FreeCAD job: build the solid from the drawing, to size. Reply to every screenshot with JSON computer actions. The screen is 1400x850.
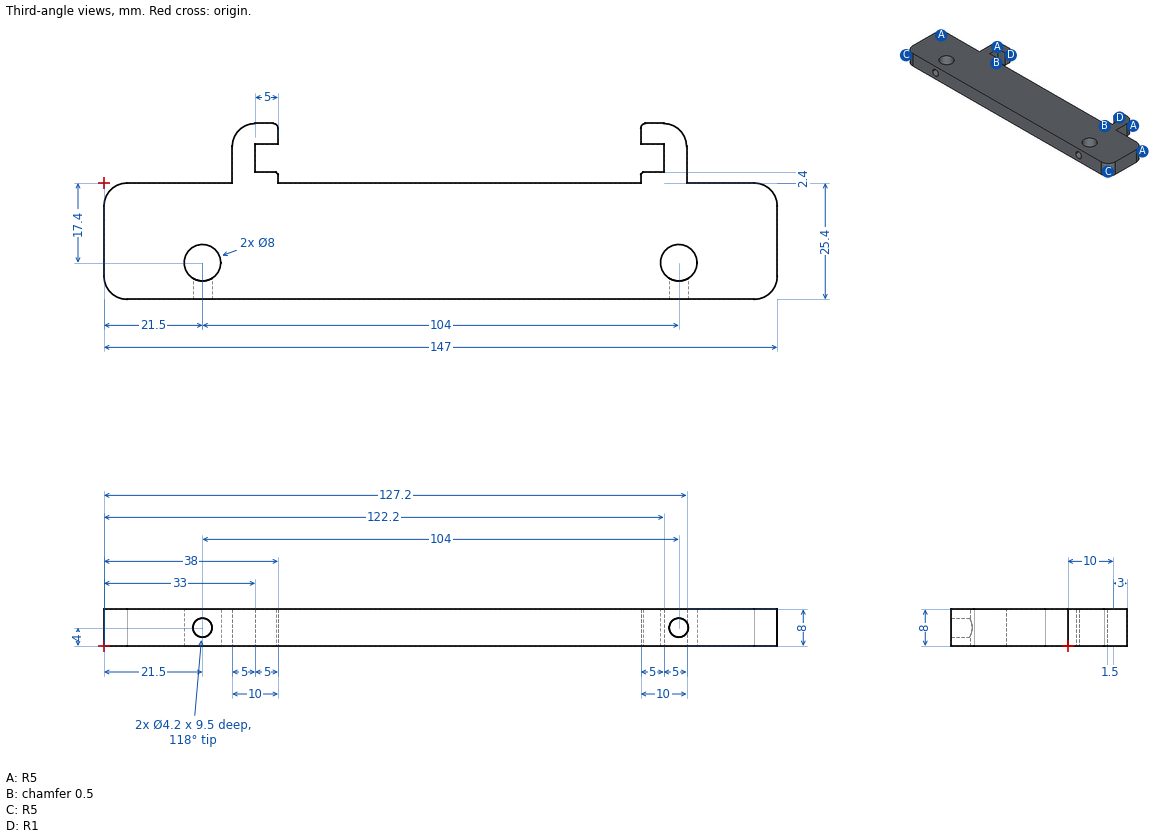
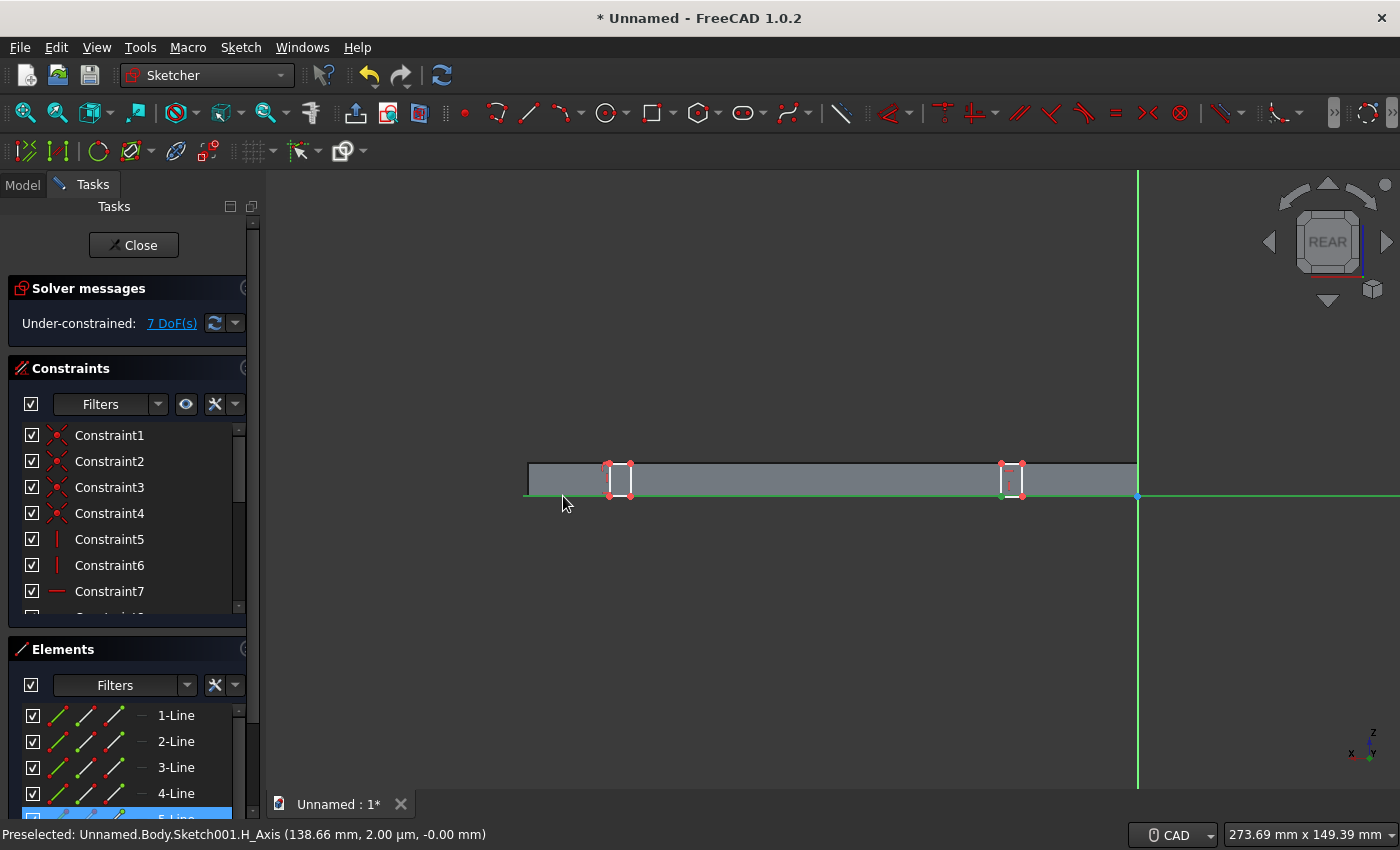
{"action": "left_click", "coordinate": [944, 114]}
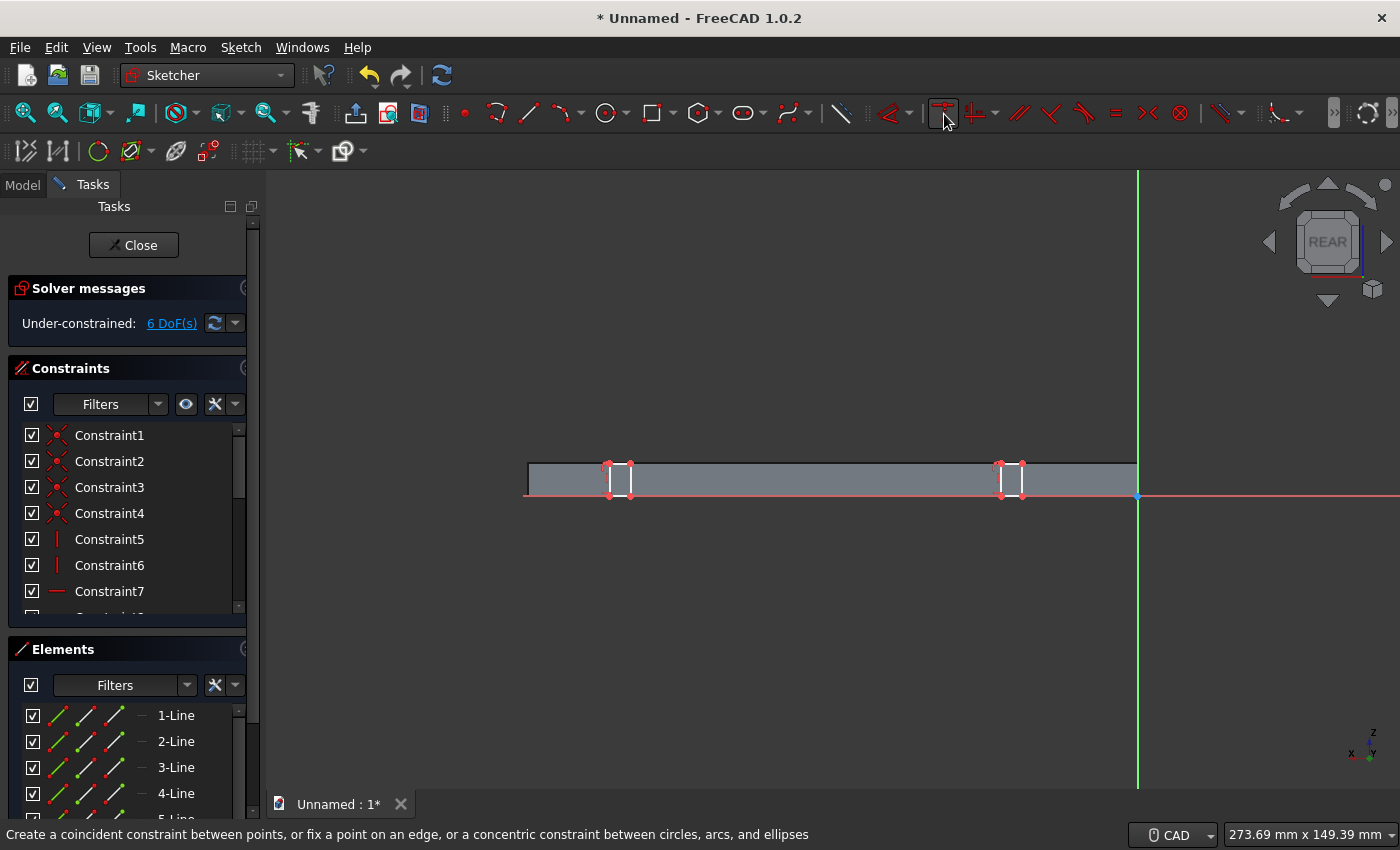
{"action": "left_click", "coordinate": [888, 114]}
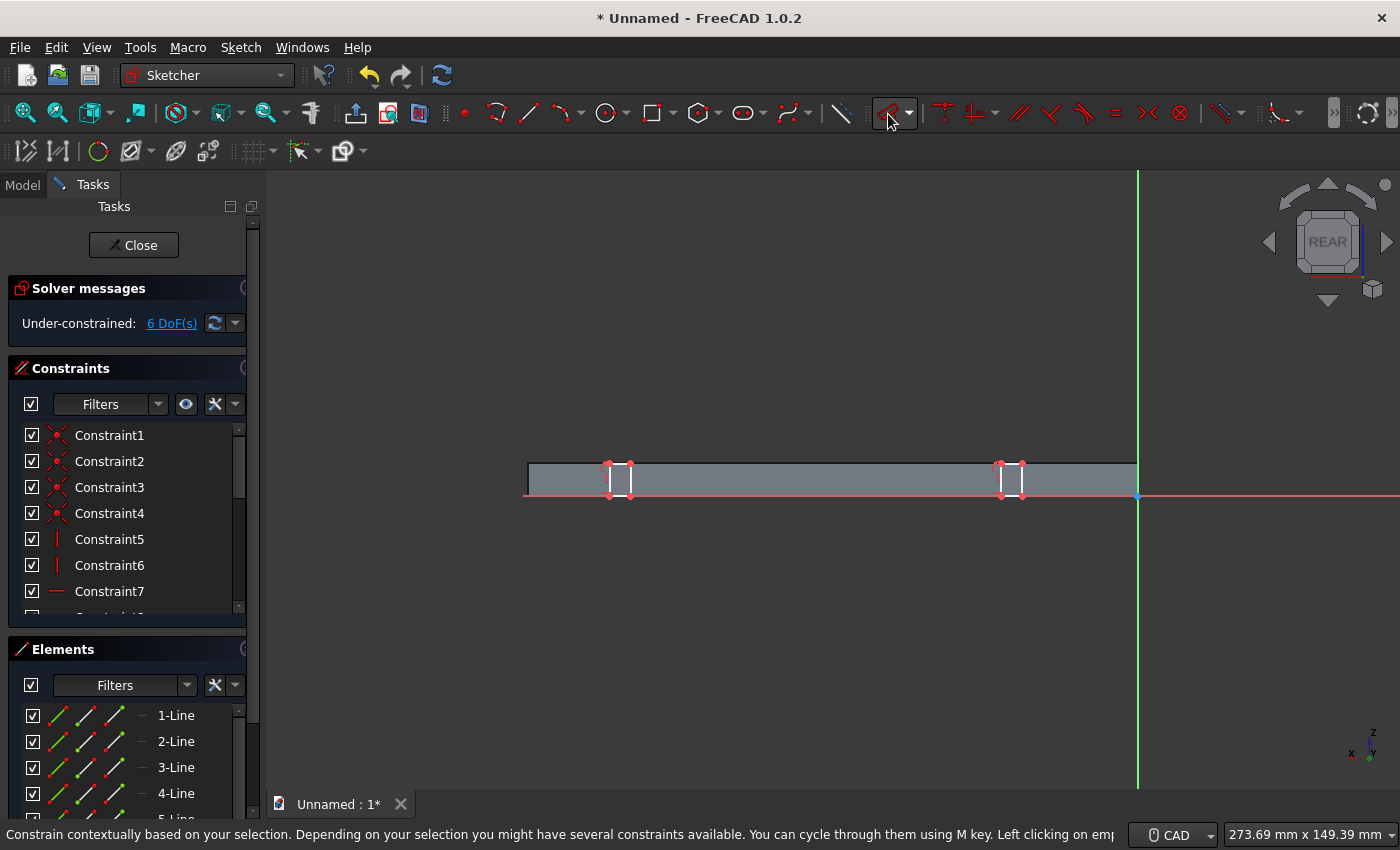
{"action": "scroll", "coordinate": [610, 474], "scroll_direction": "up", "scroll_amount": 2}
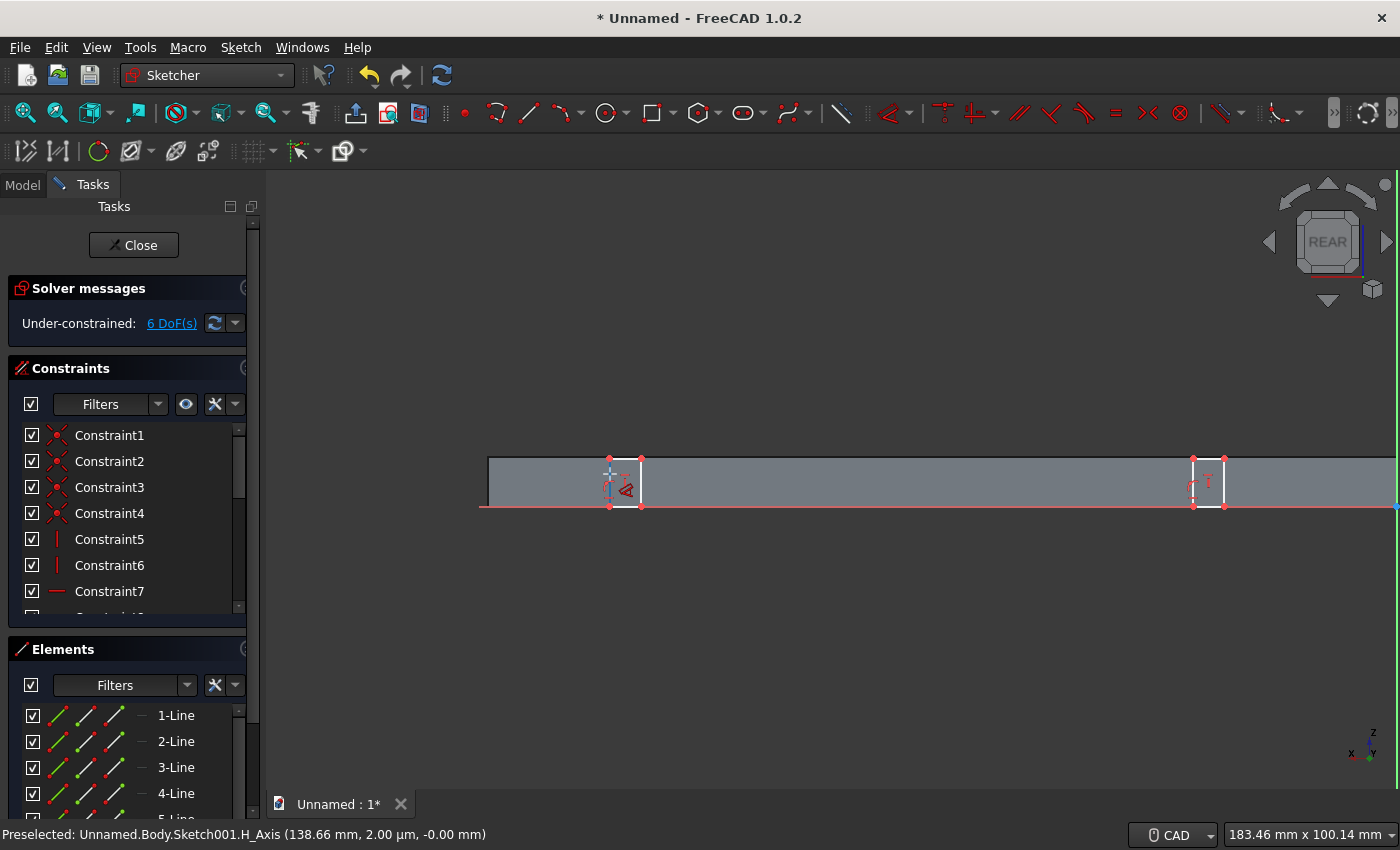
{"action": "left_click", "coordinate": [610, 473]}
{"action": "left_click", "coordinate": [576, 483]}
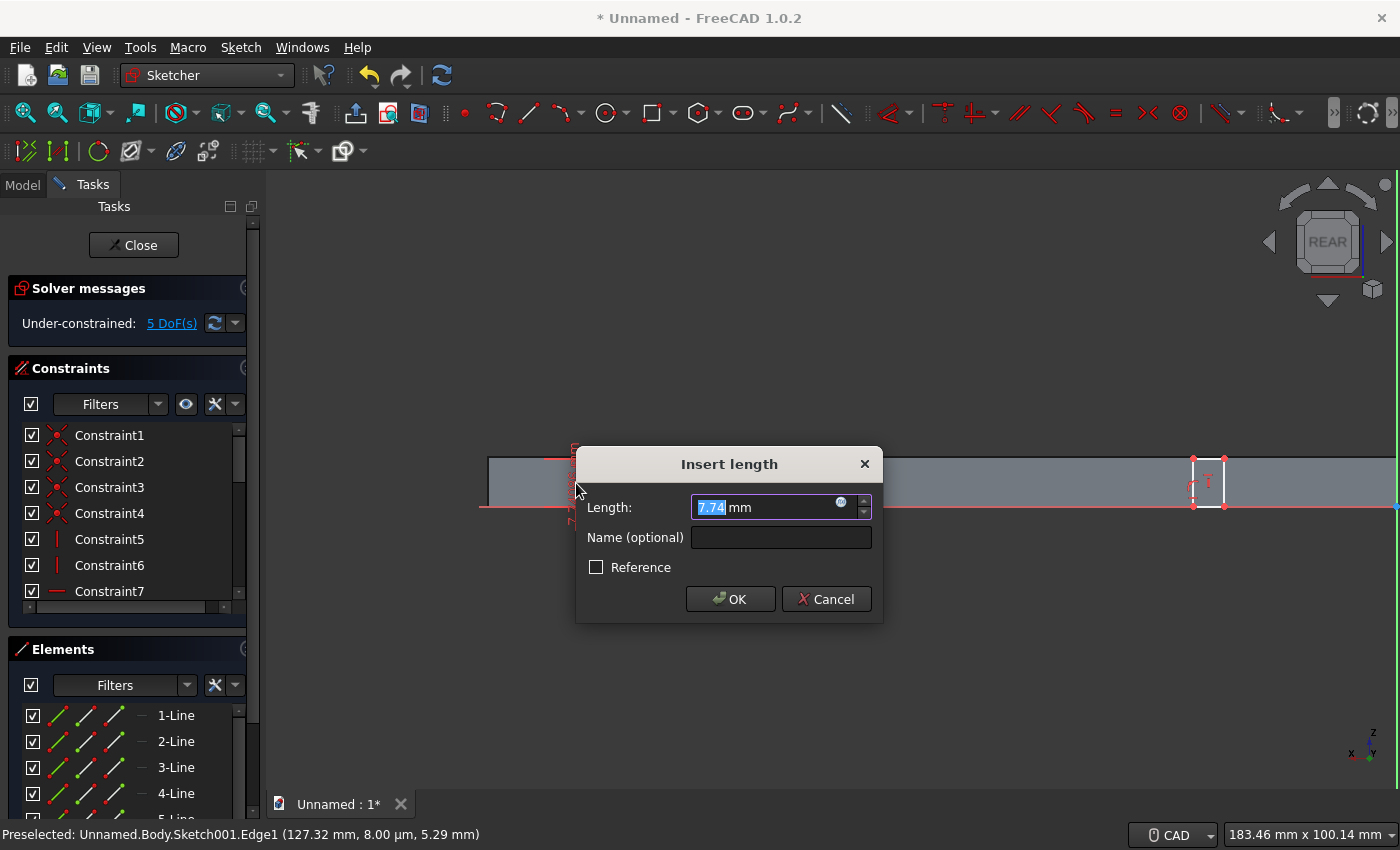
{"action": "type", "text": "8"}
{"action": "key", "text": "Return"}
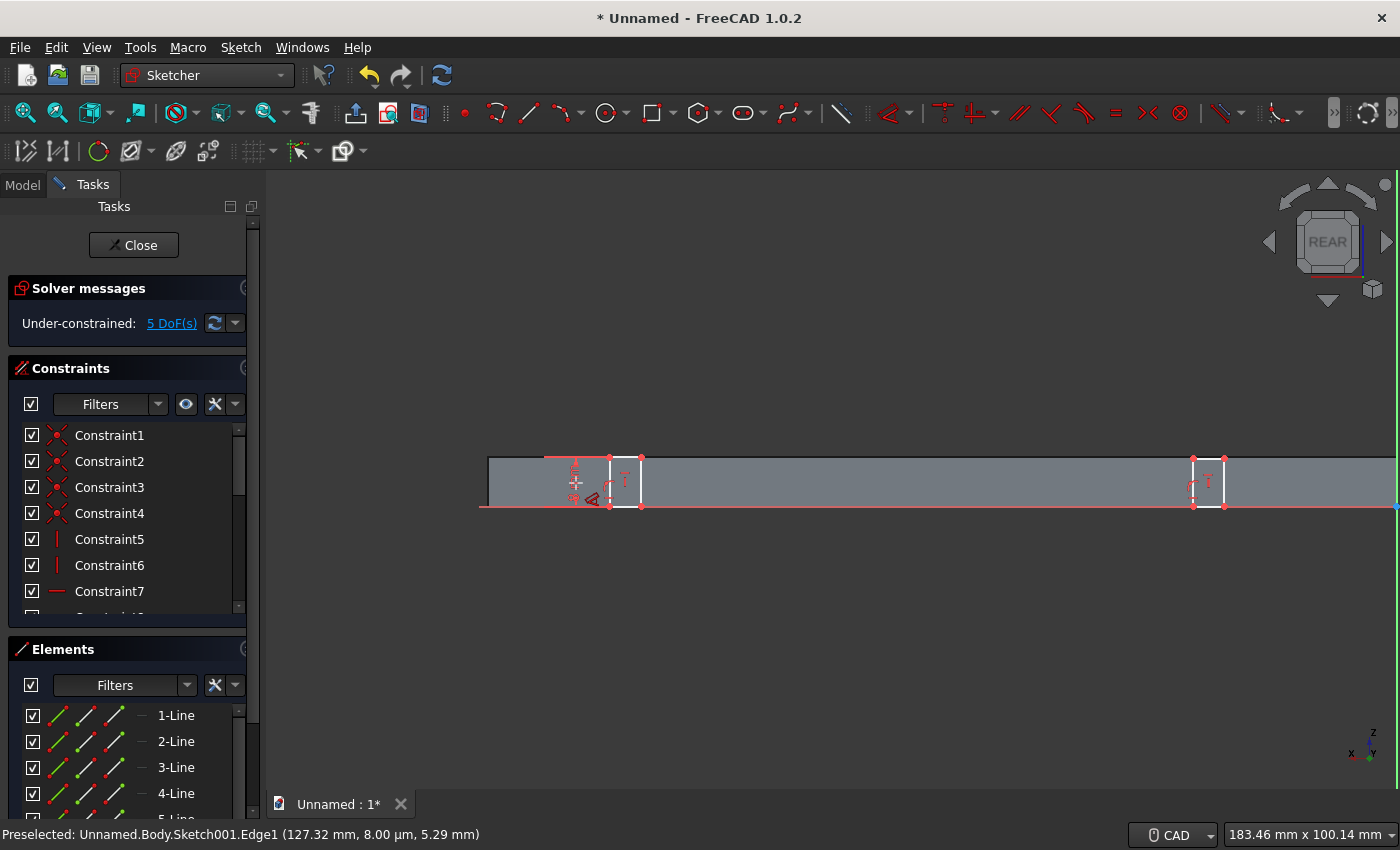
{"action": "scroll", "coordinate": [619, 507], "scroll_direction": "up", "scroll_amount": 2}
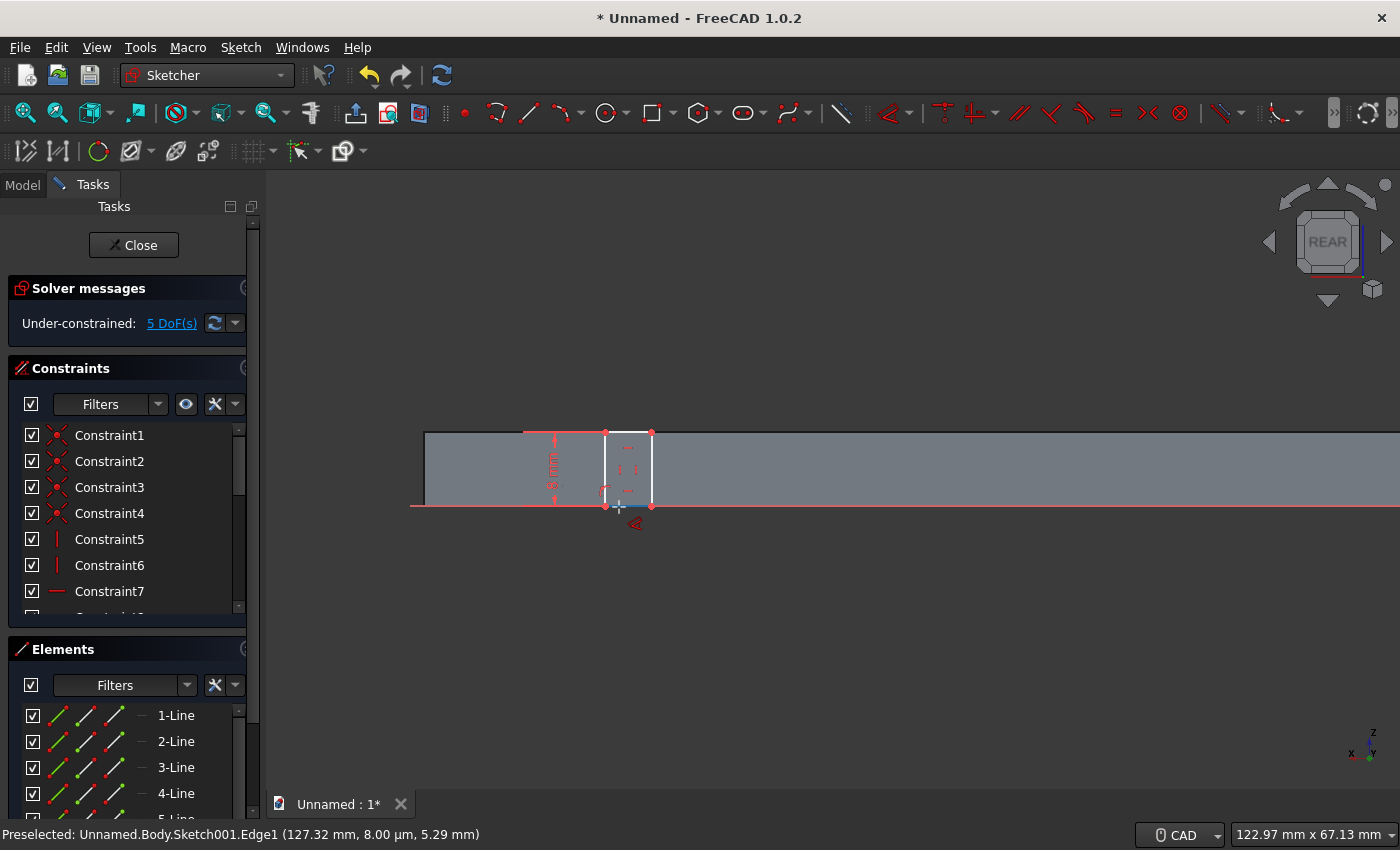
{"action": "left_click", "coordinate": [619, 506]}
{"action": "left_click", "coordinate": [629, 540]}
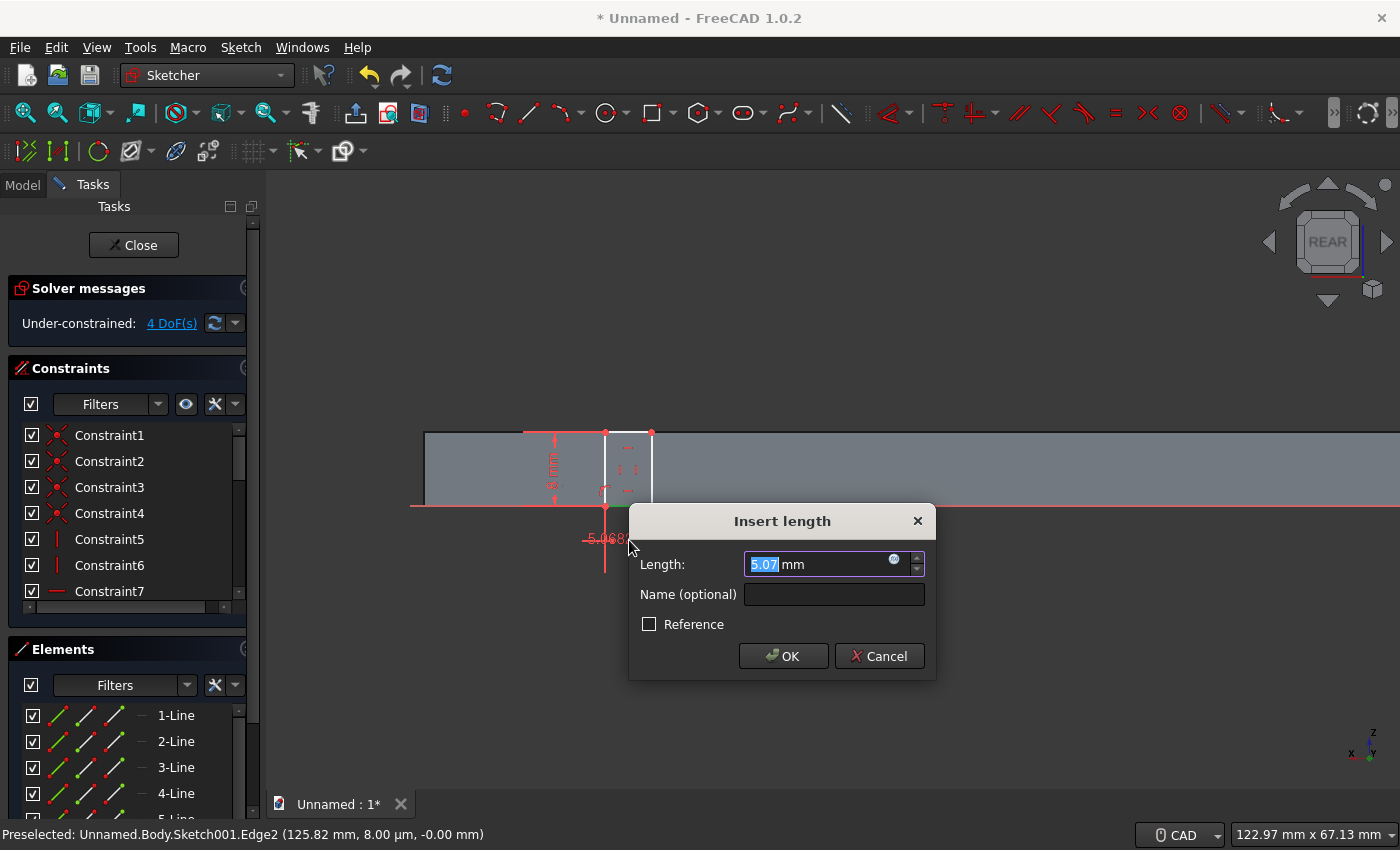
{"action": "type", "text": "5"}
{"action": "key", "text": "Return"}